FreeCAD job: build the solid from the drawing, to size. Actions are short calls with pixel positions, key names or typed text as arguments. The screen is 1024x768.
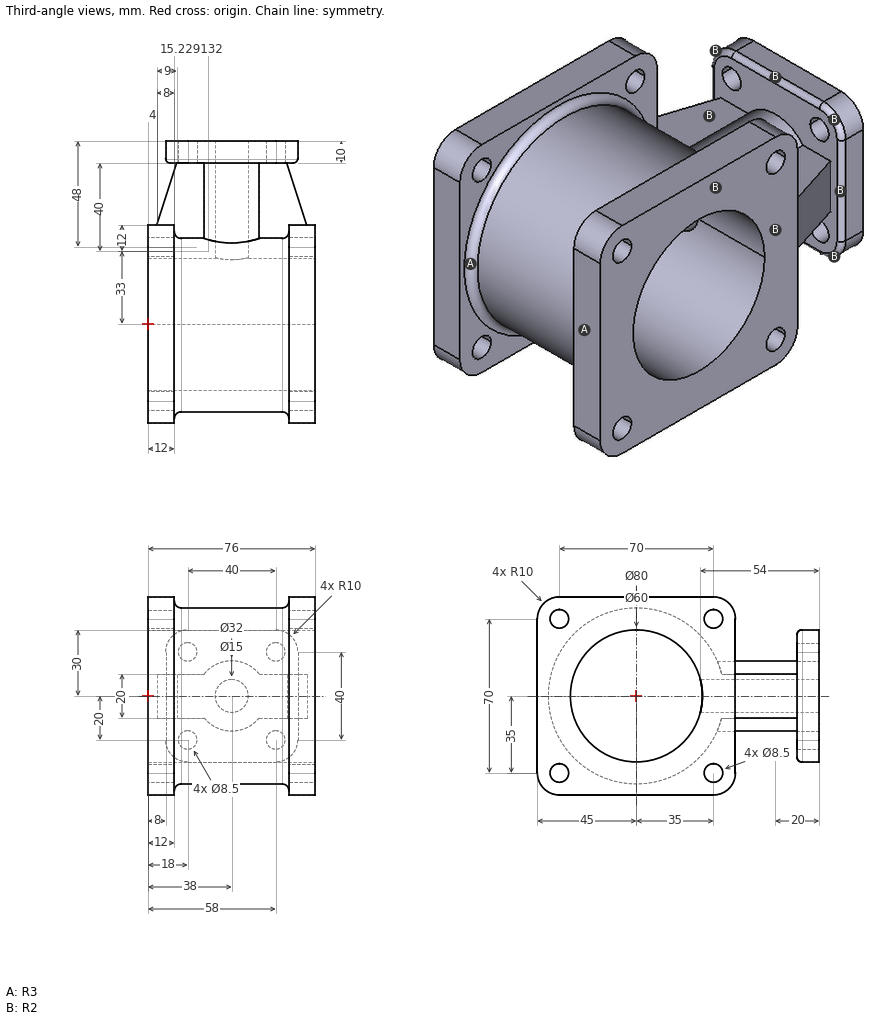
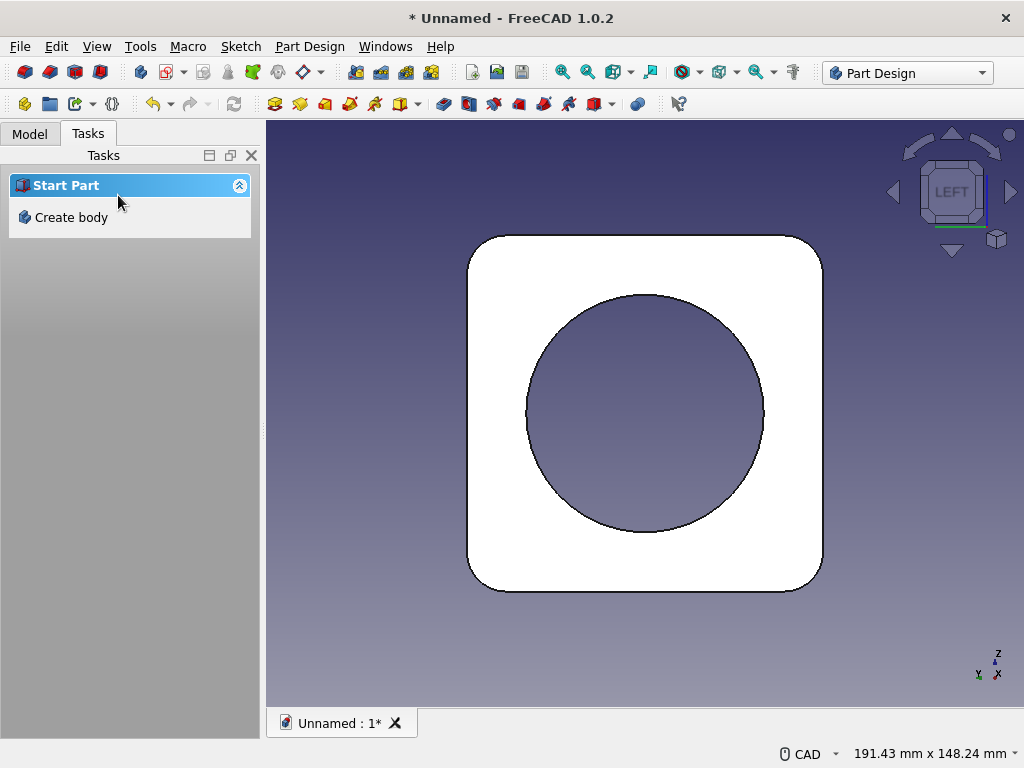
click(166, 72)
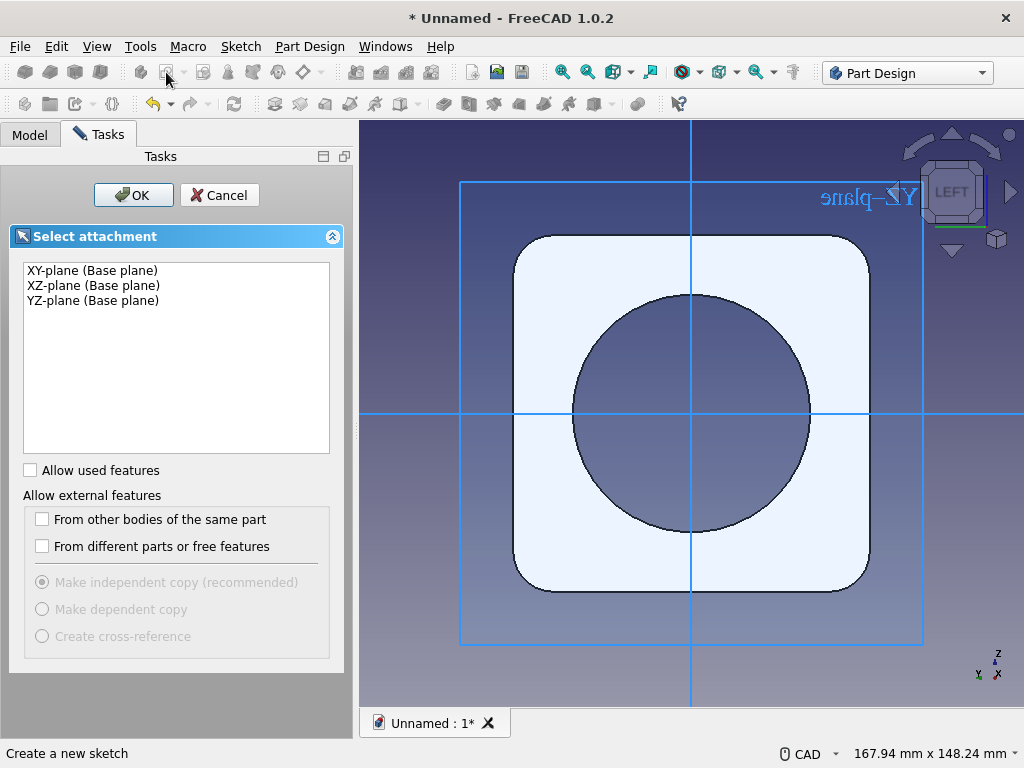
click(84, 300)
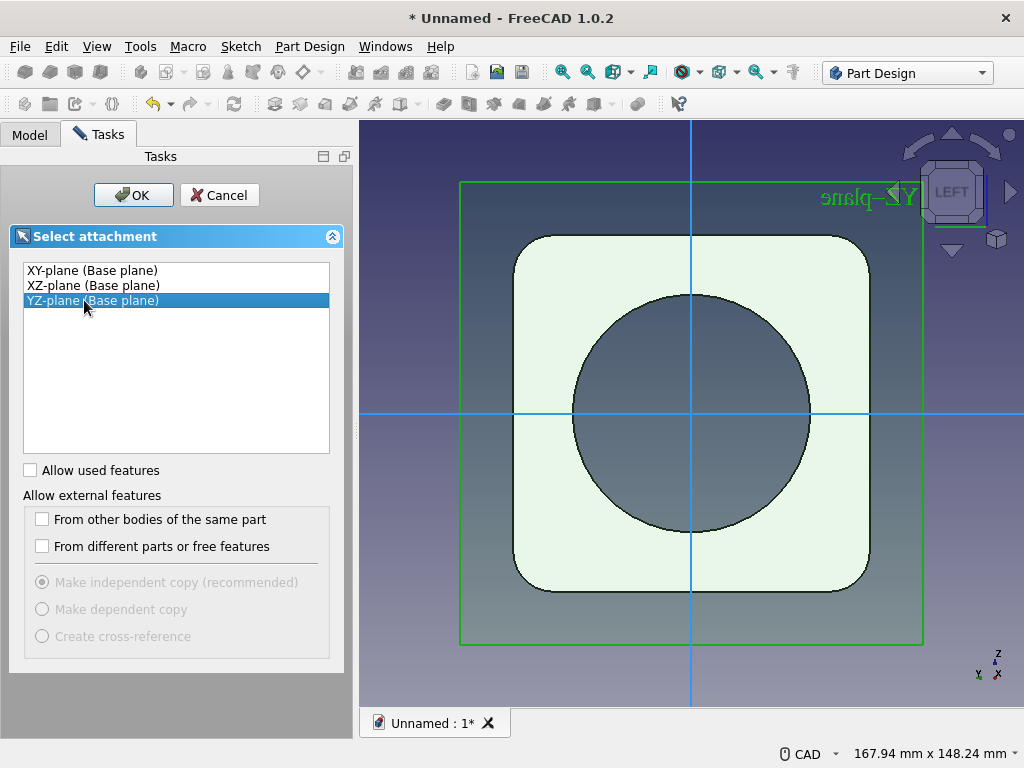
click(134, 195)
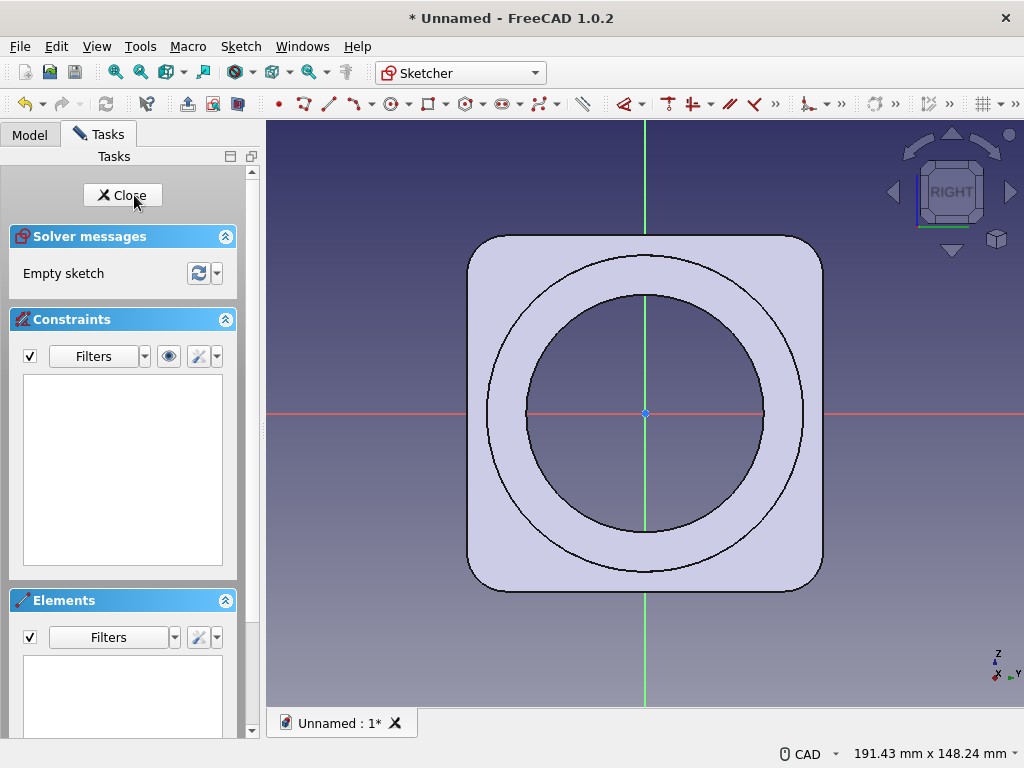
key(q)
key(s)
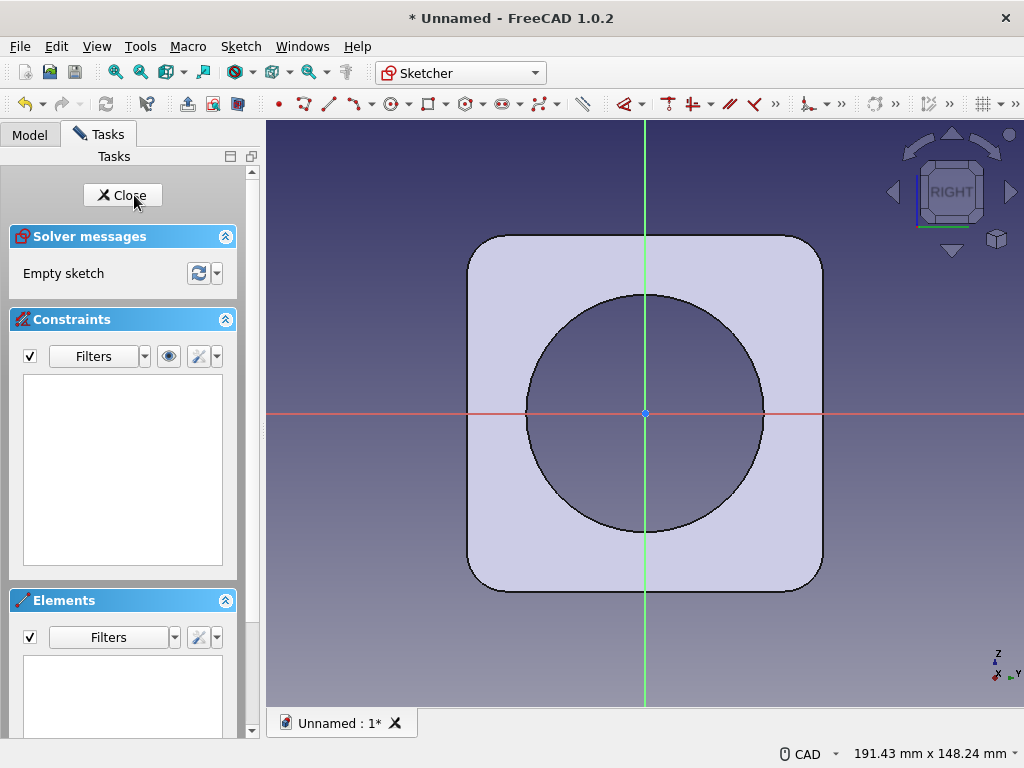
click(390, 104)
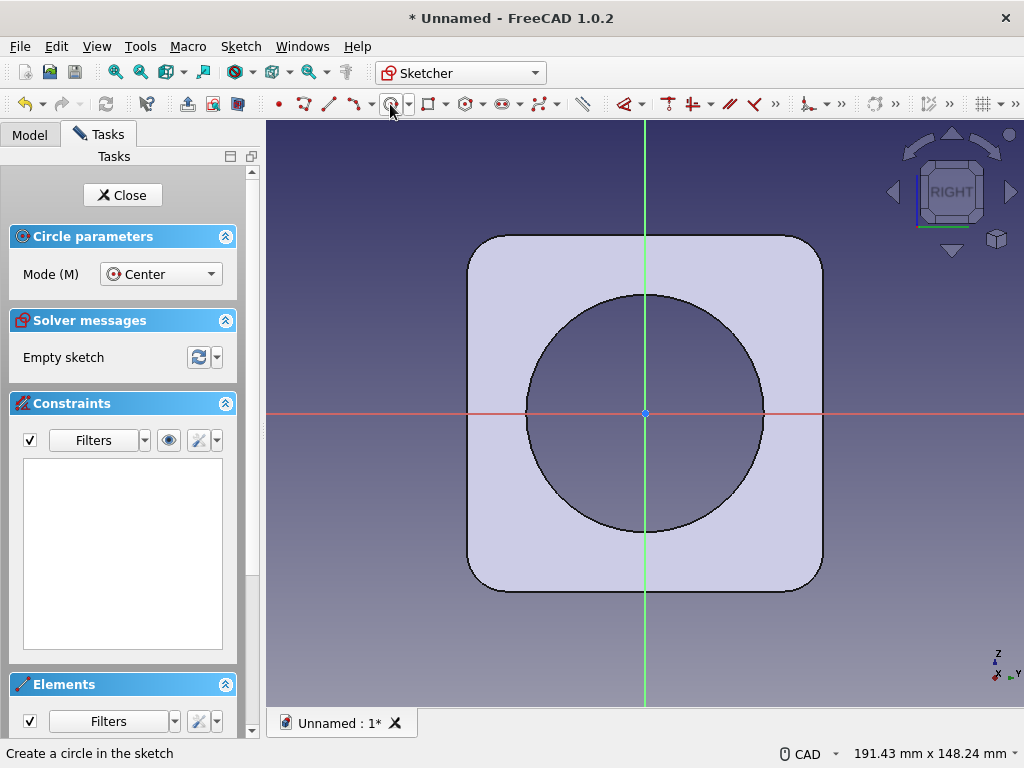
scroll(784, 552, up, 2)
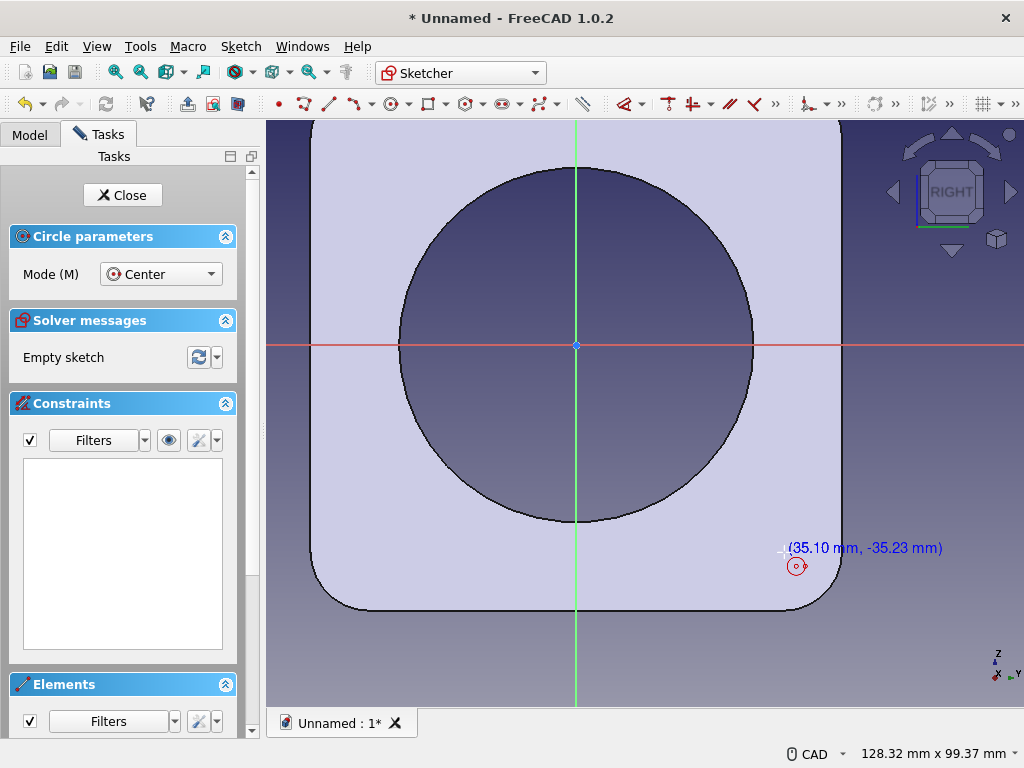
click(783, 552)
click(801, 534)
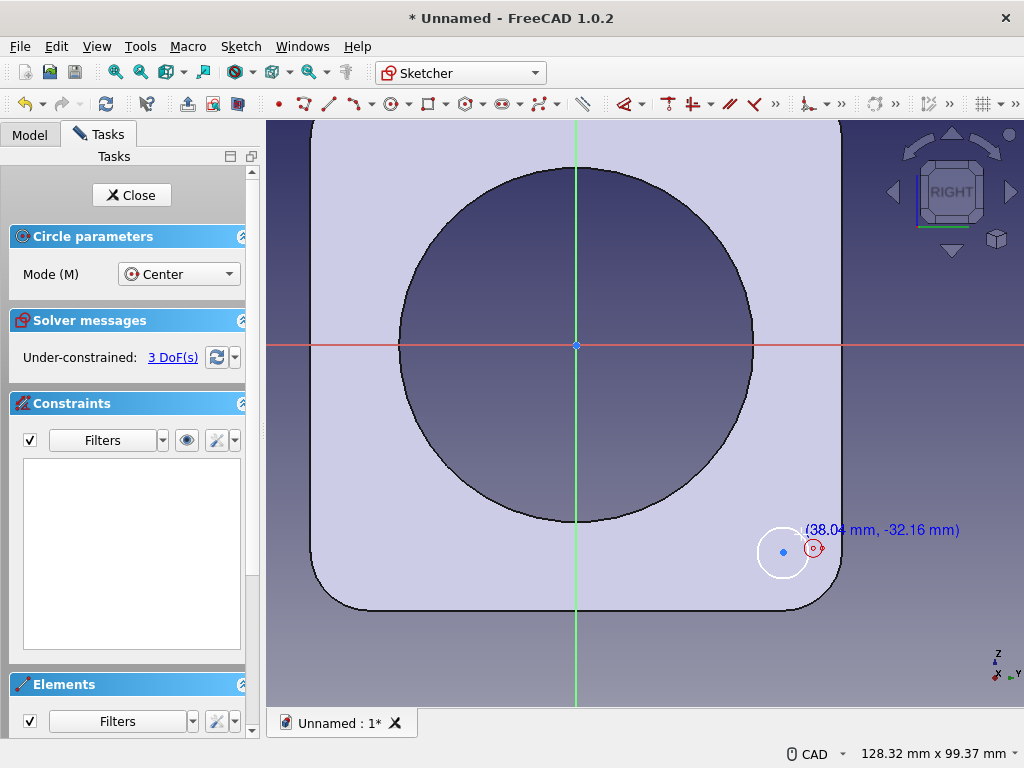
scroll(577, 679, down, 1)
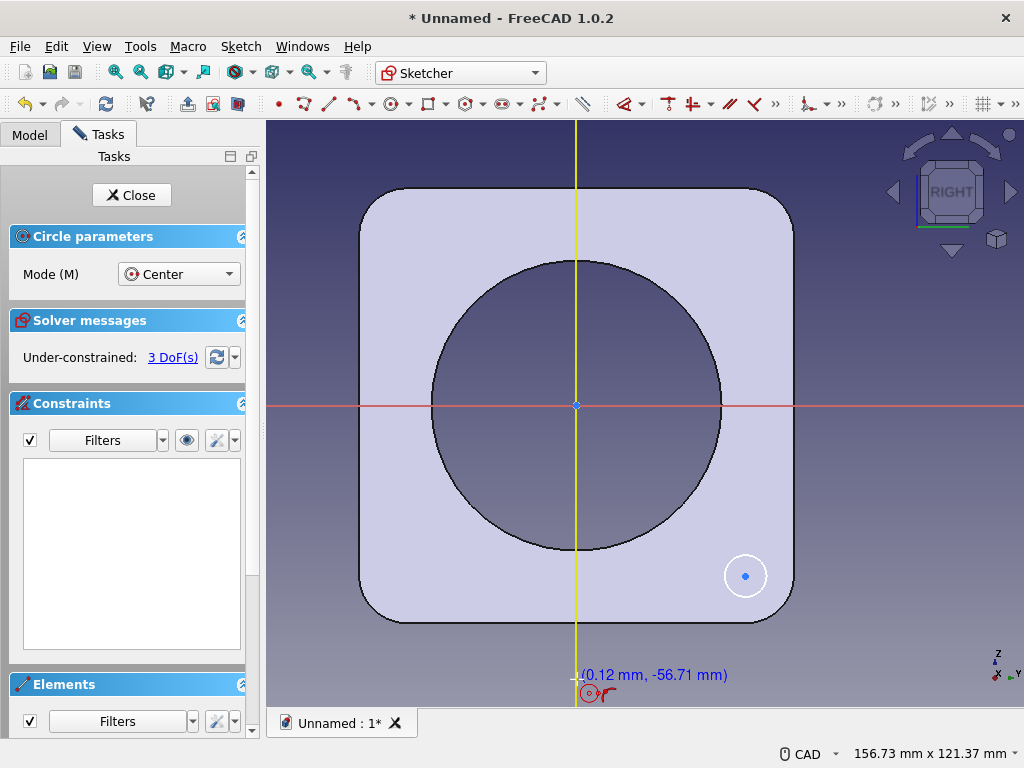
click(746, 236)
click(760, 222)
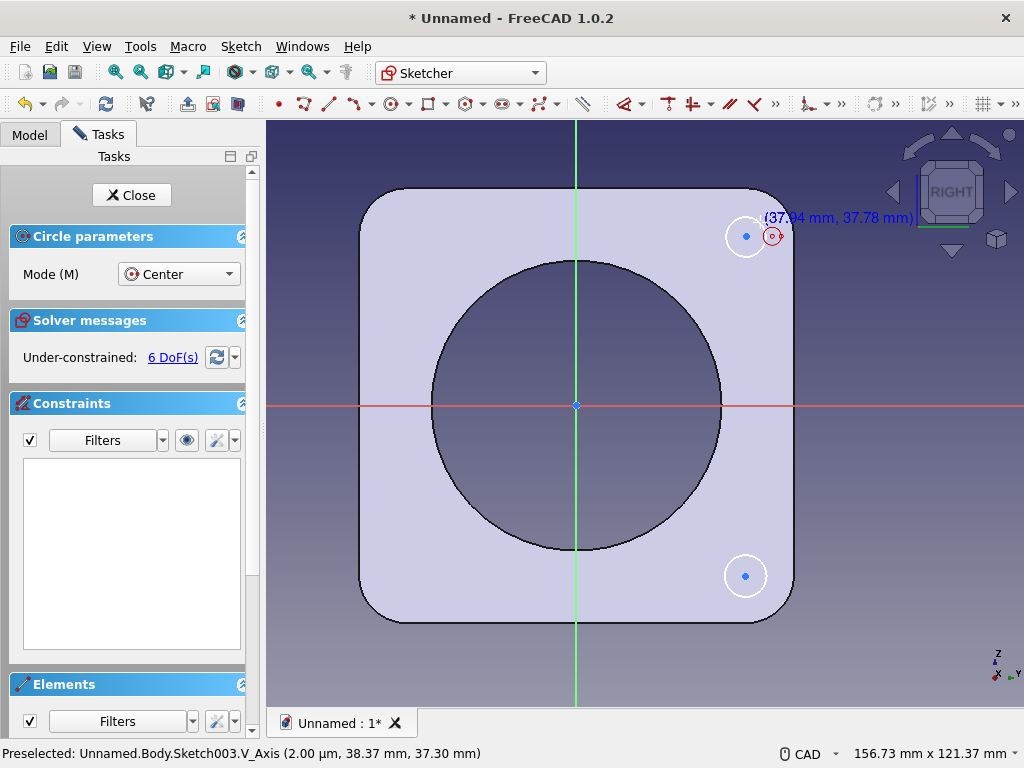
click(407, 575)
click(422, 560)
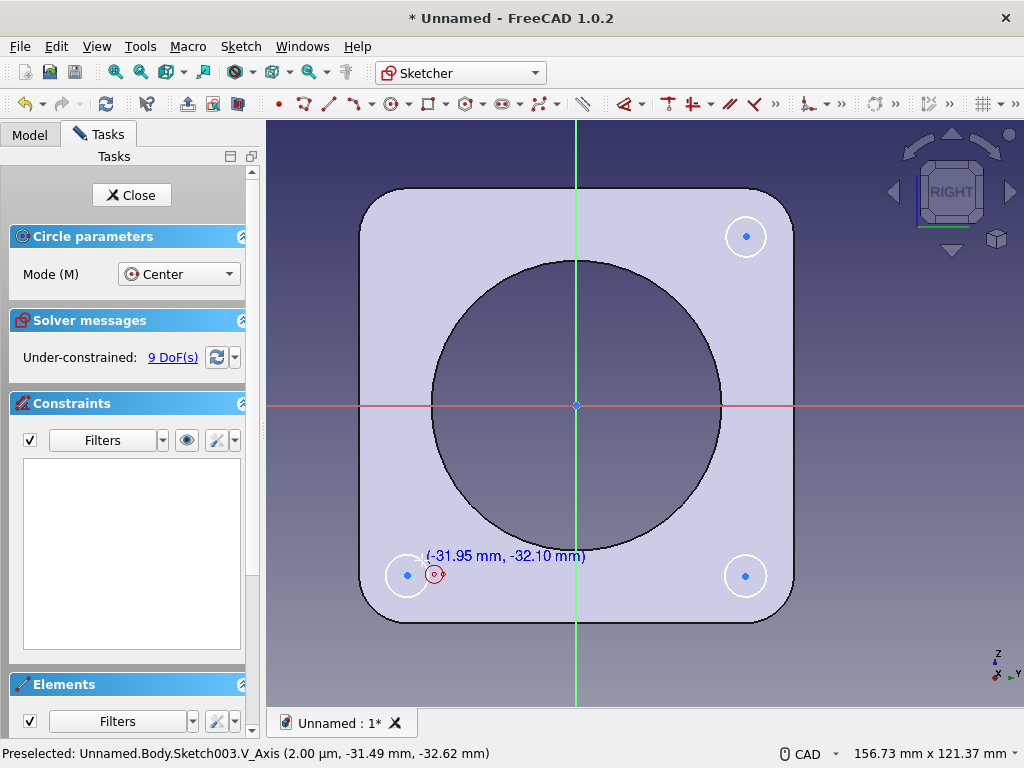
click(407, 236)
click(422, 222)
key(Escape)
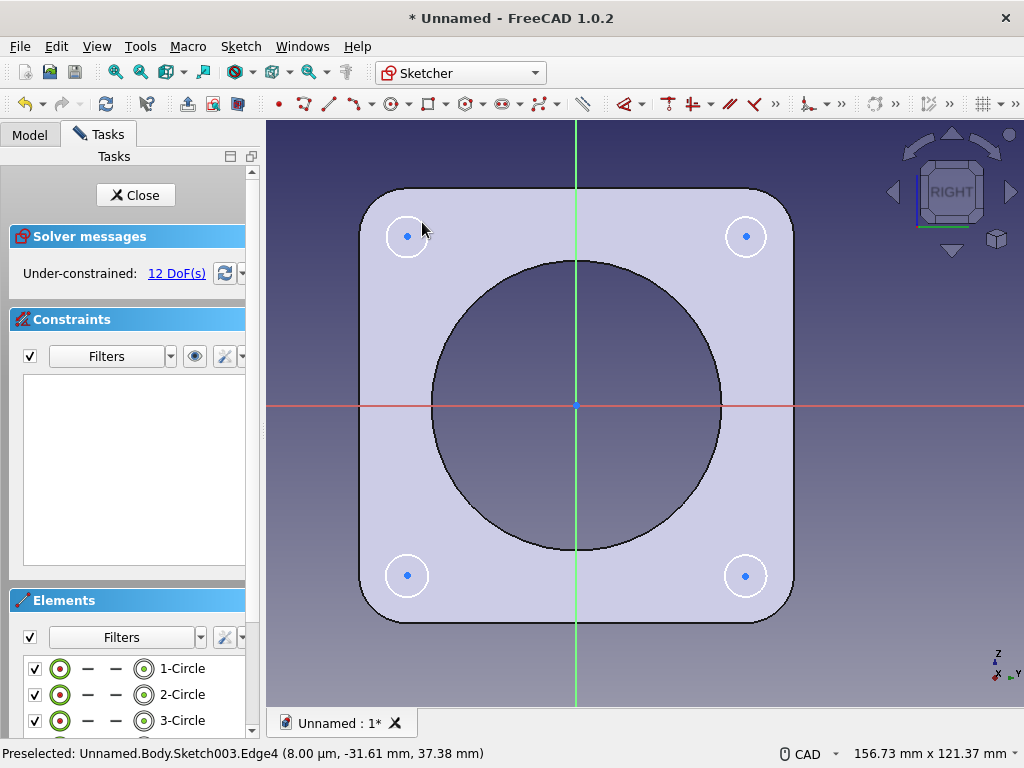
click(760, 561)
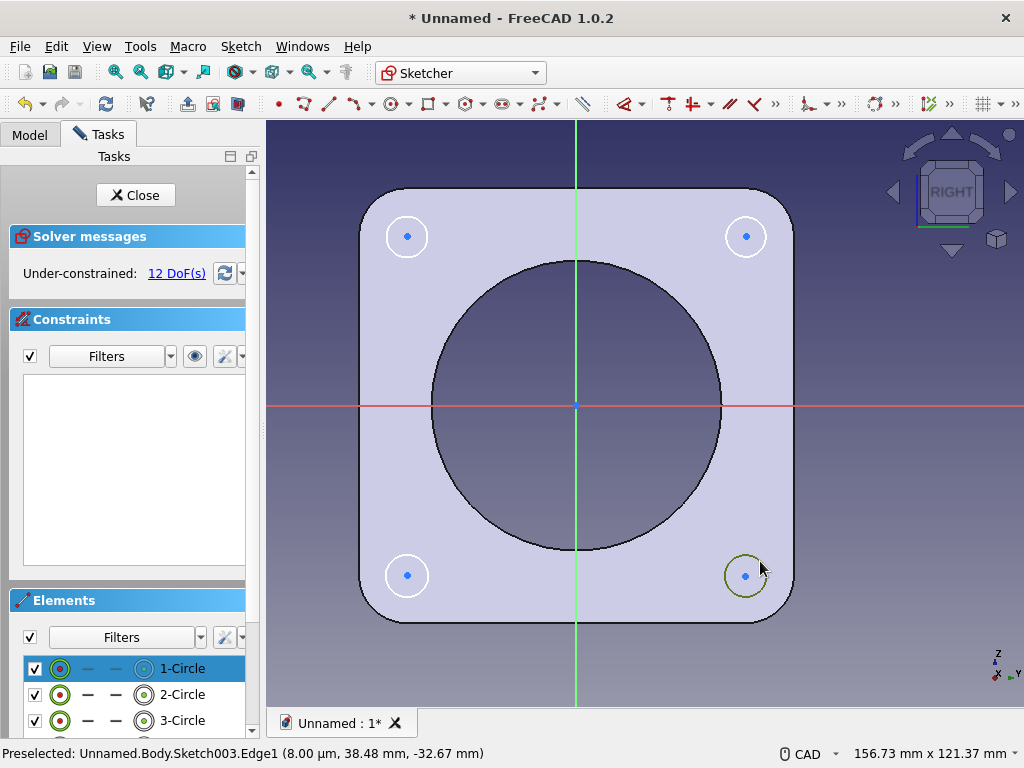
click(760, 223)